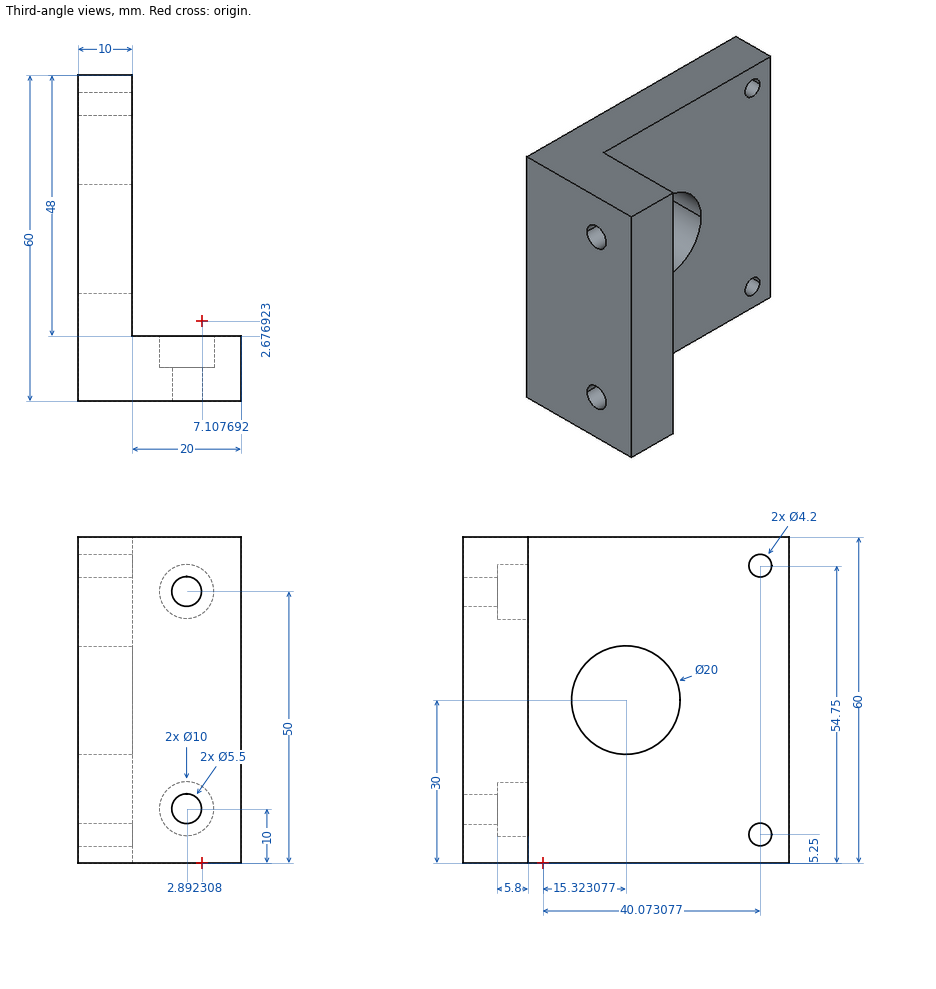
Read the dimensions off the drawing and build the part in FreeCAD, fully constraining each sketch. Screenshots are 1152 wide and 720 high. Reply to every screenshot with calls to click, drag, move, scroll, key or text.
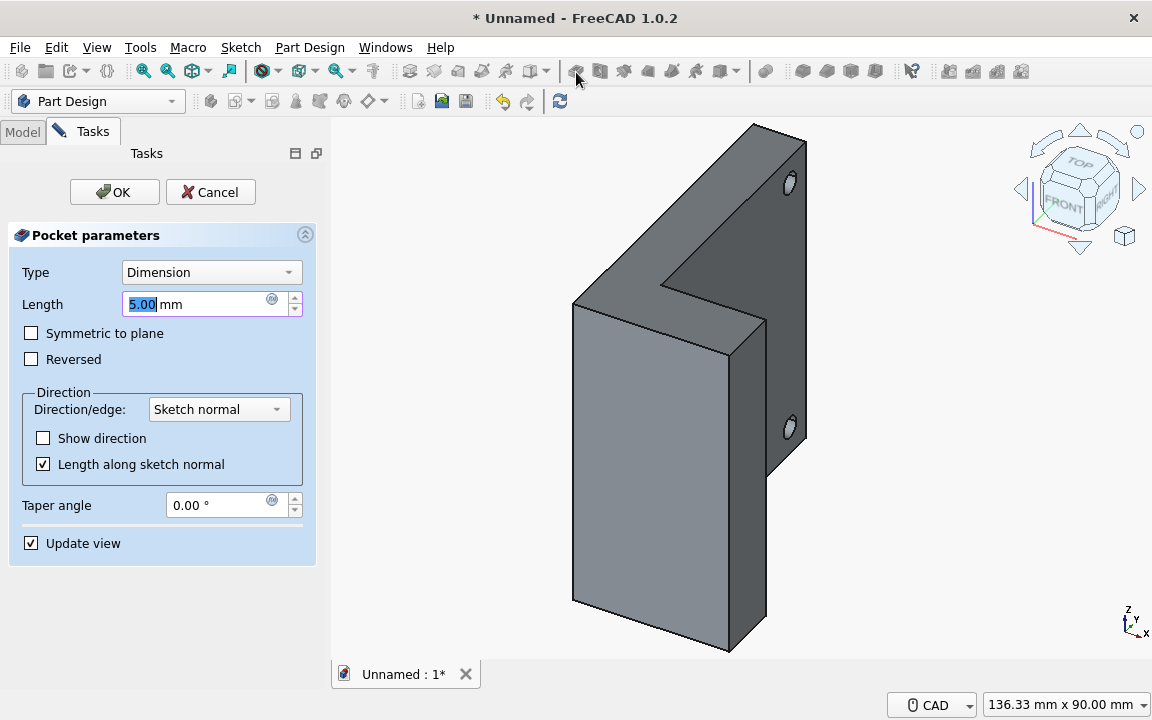
click(212, 272)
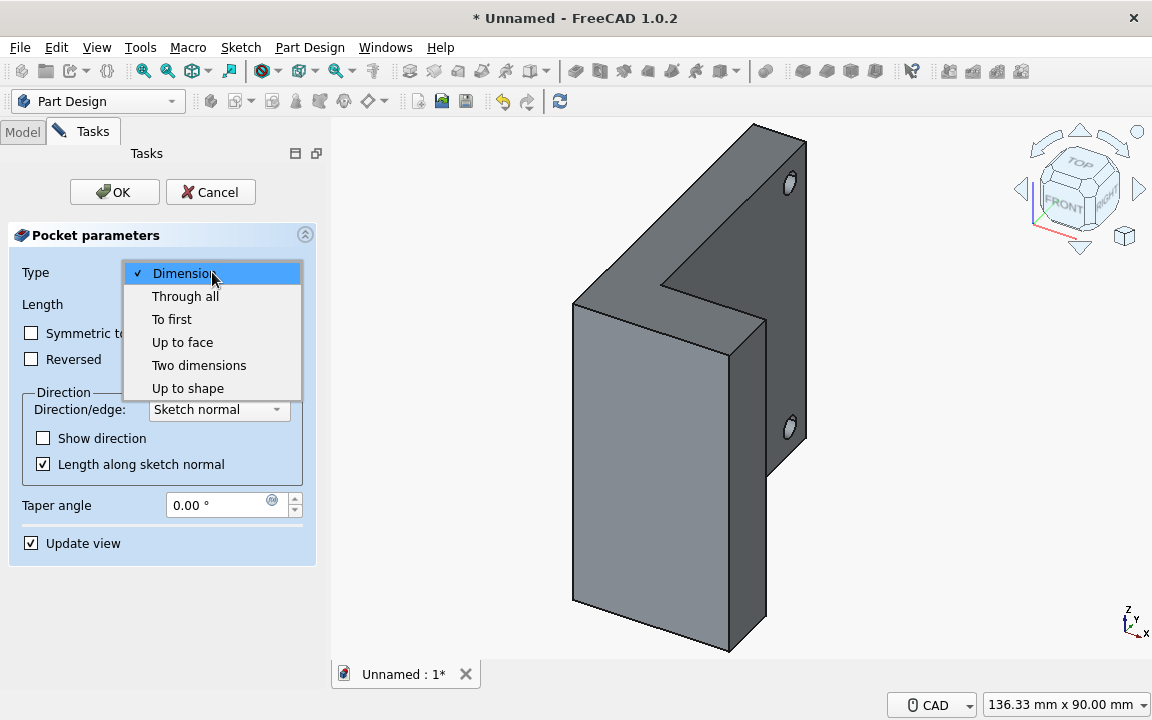
click(212, 296)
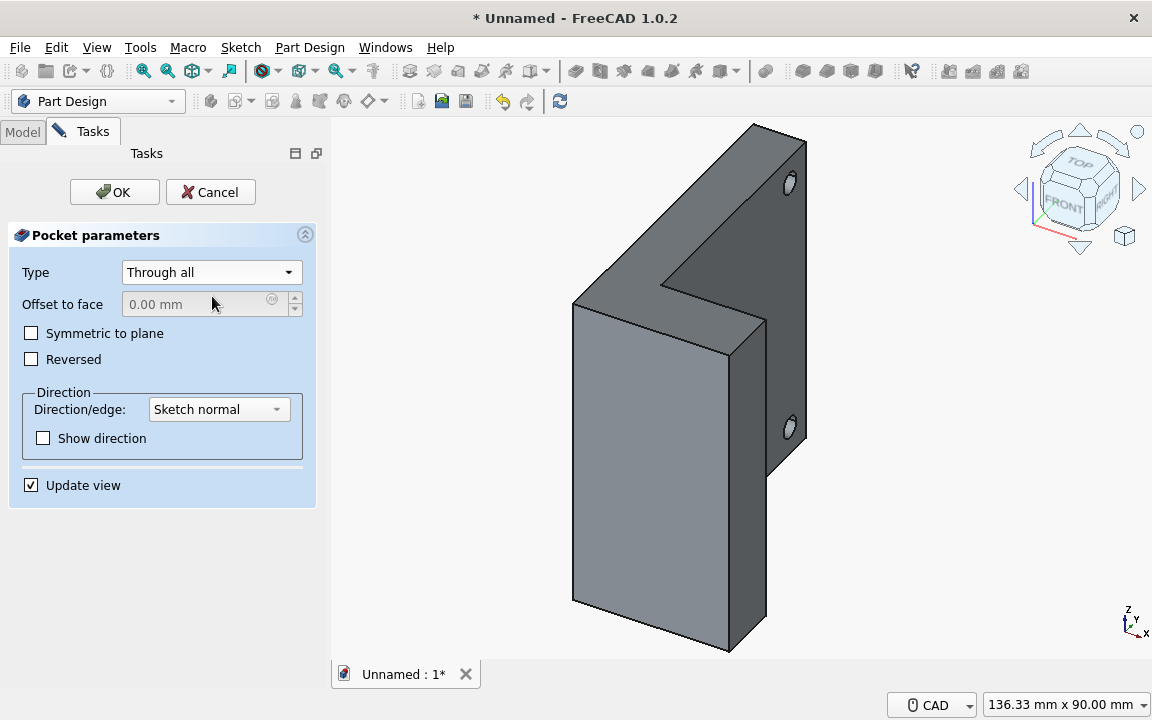
click(115, 192)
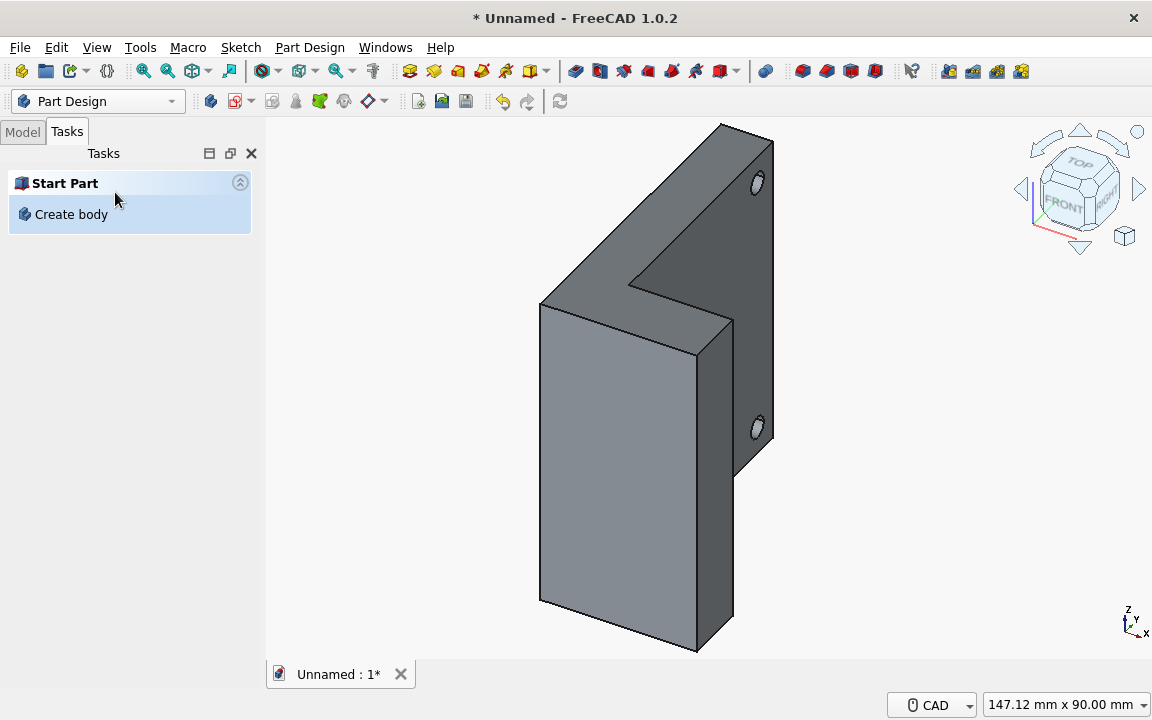
key(4)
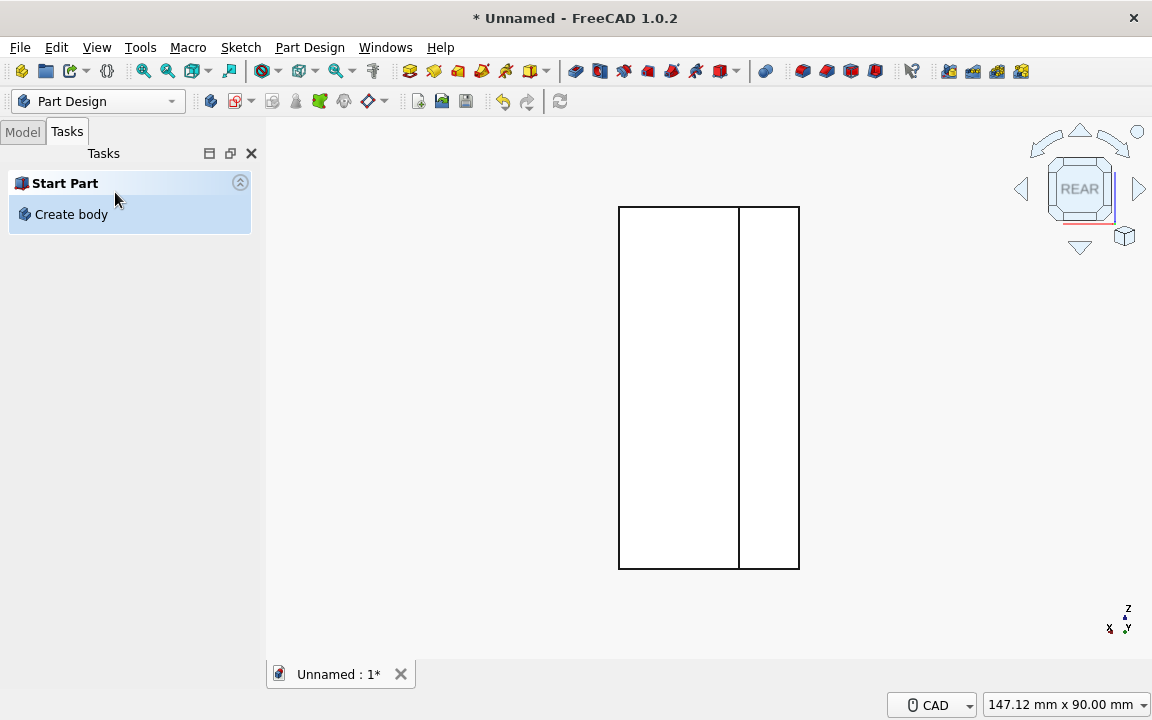
click(679, 284)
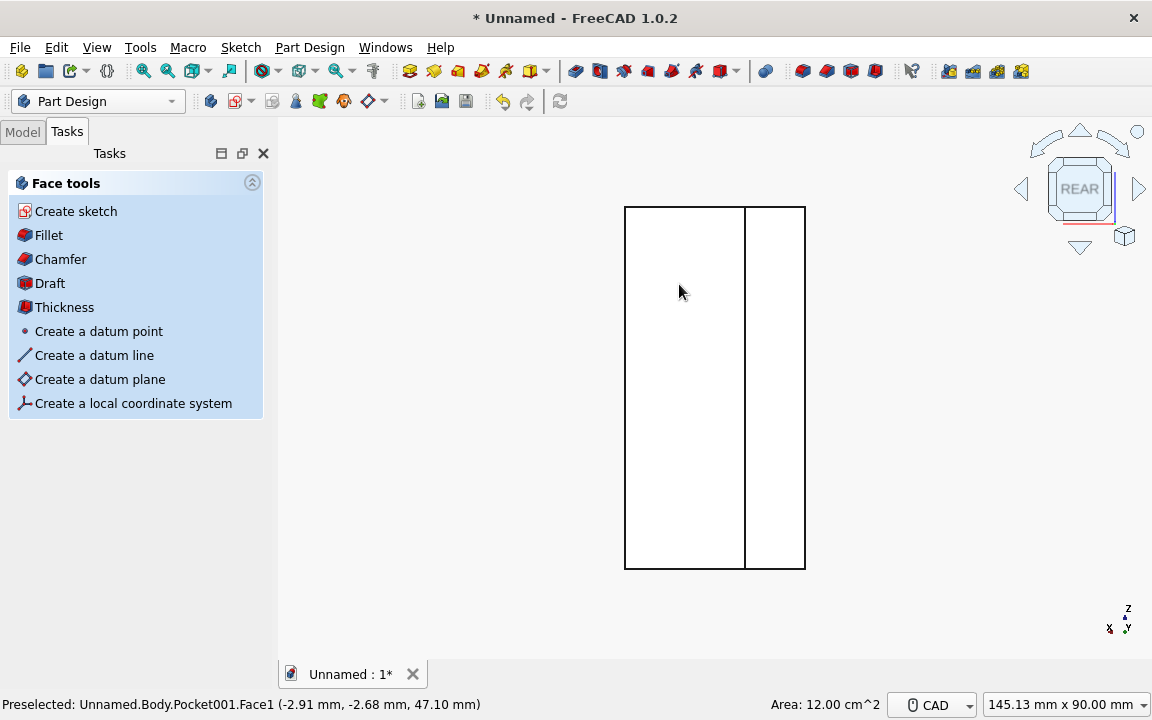
click(236, 102)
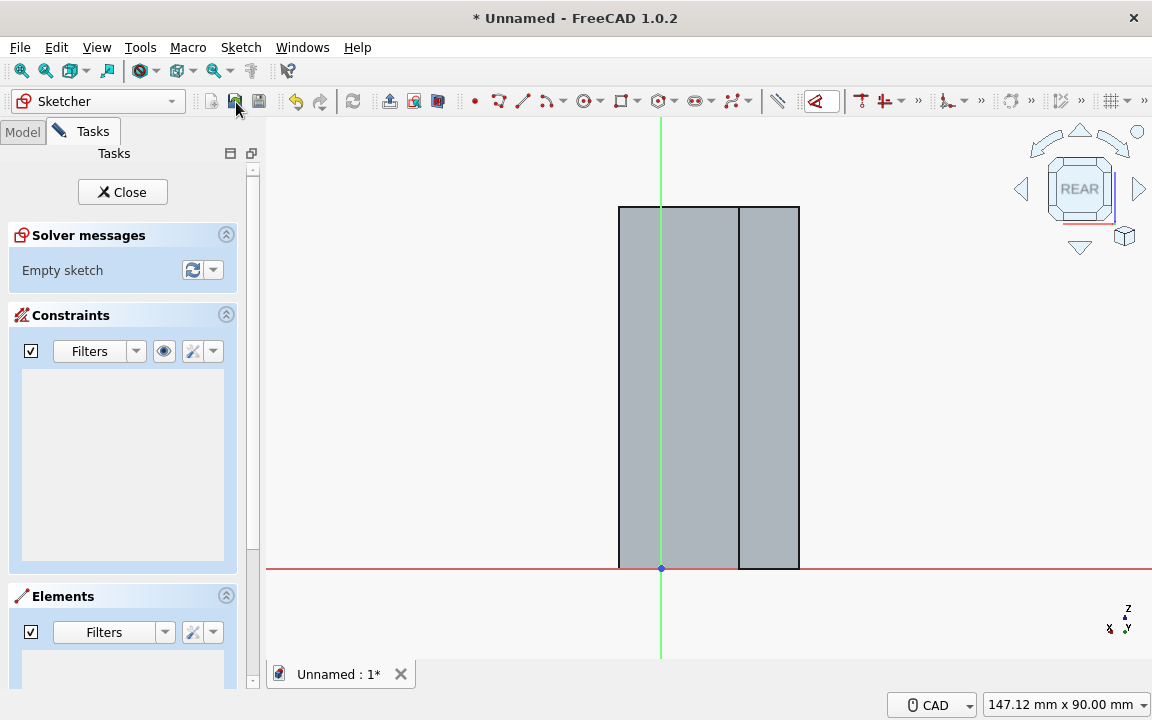
click(438, 102)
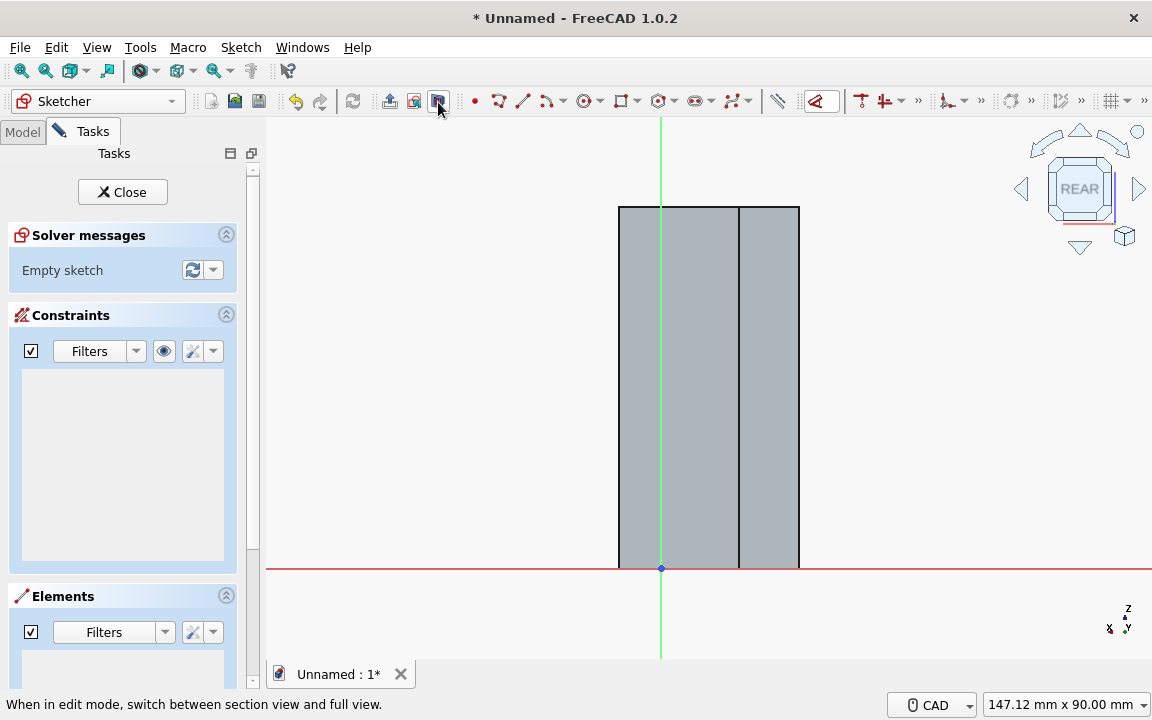
click(584, 102)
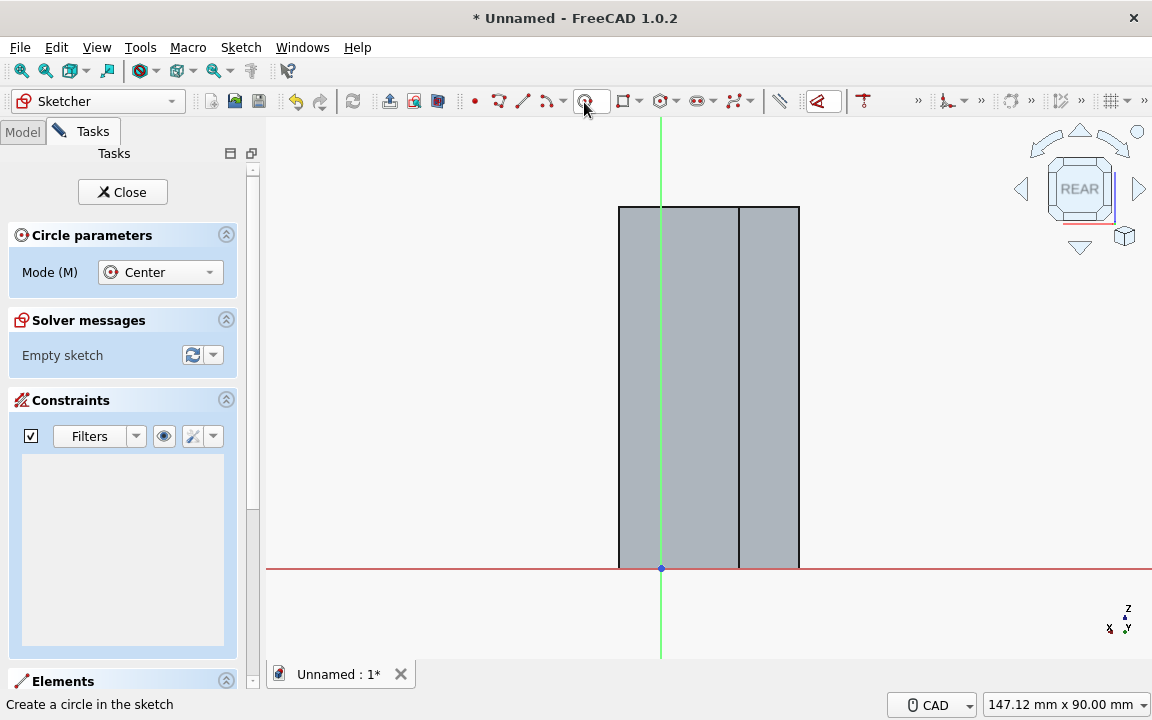
scroll(679, 508, up, 2)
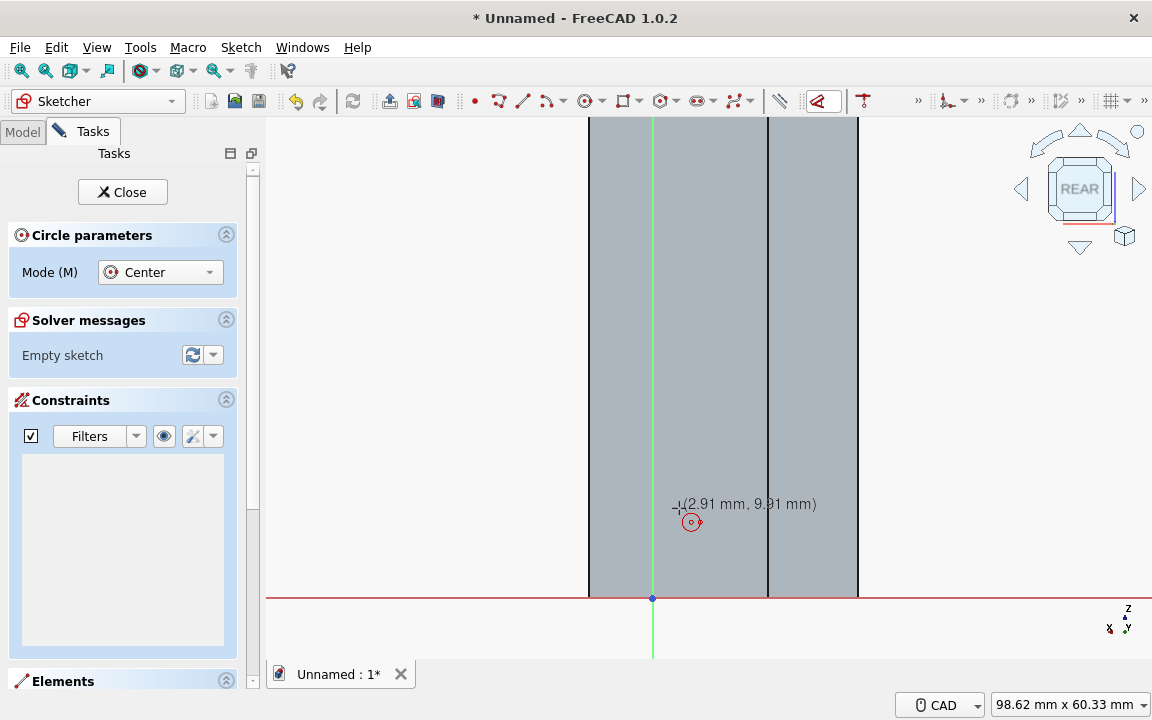
click(679, 508)
move(696, 491)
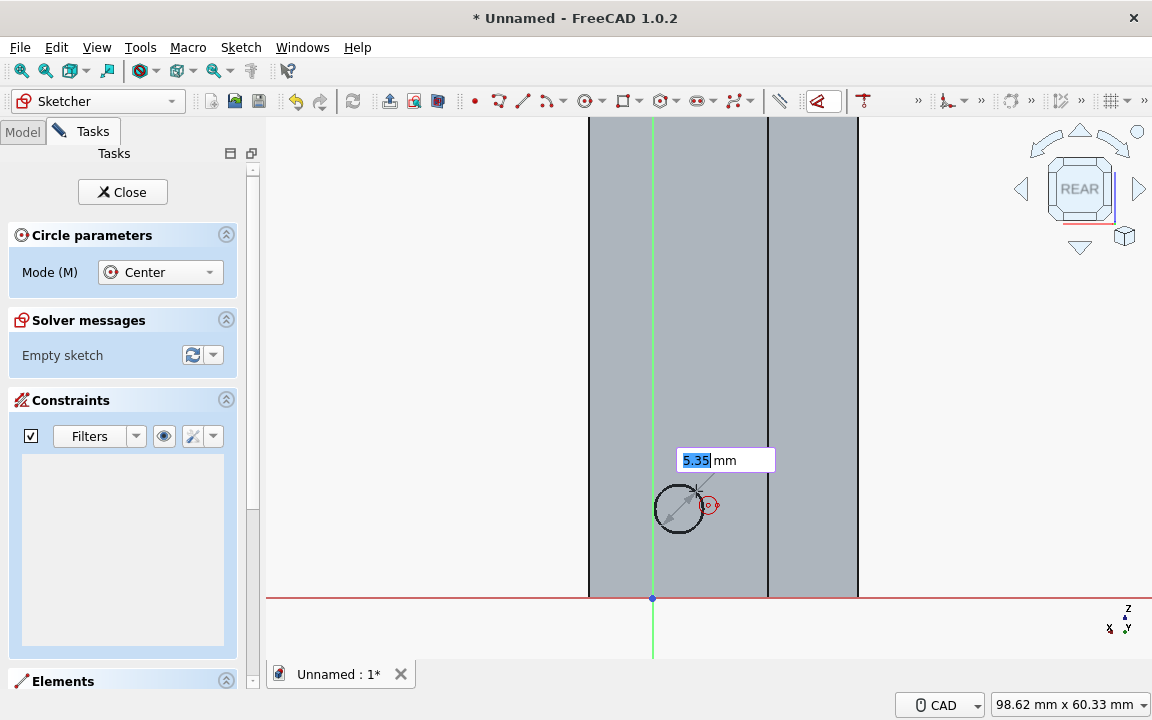
text(5.5)
key(Return)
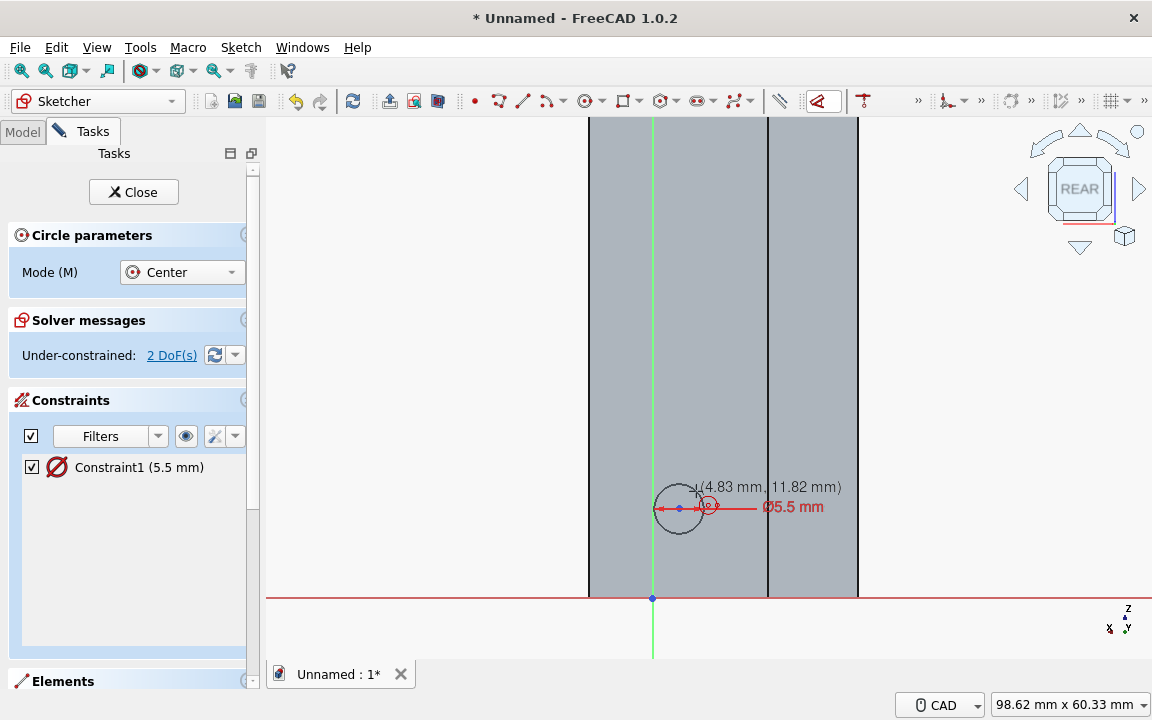
click(679, 149)